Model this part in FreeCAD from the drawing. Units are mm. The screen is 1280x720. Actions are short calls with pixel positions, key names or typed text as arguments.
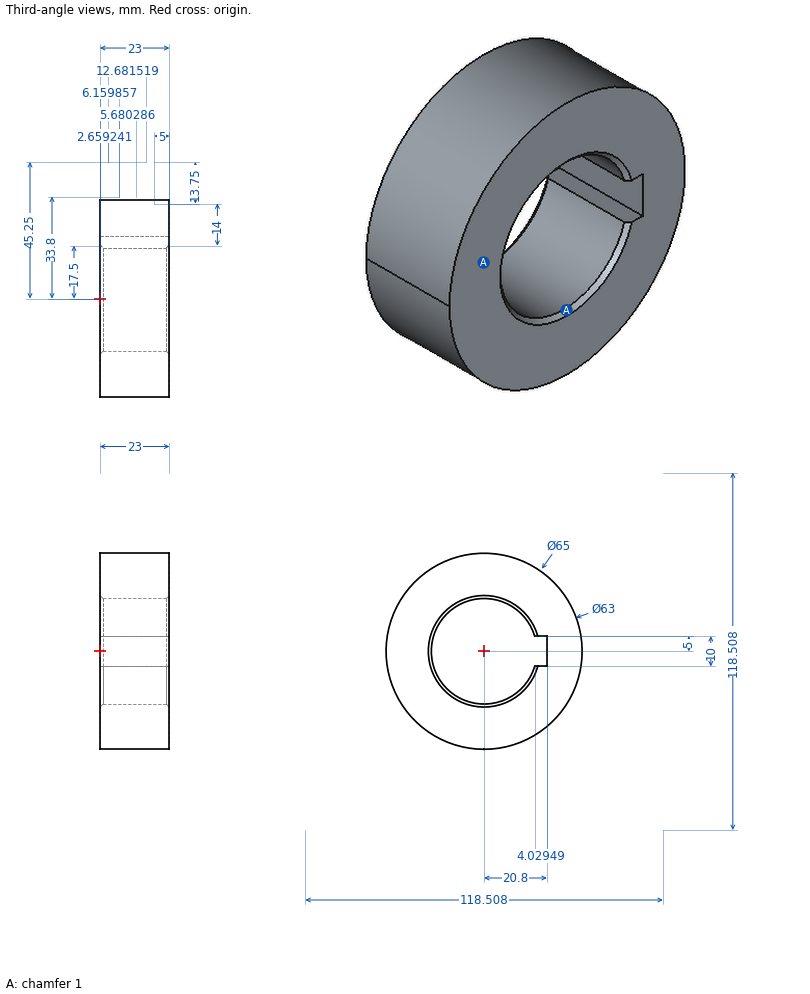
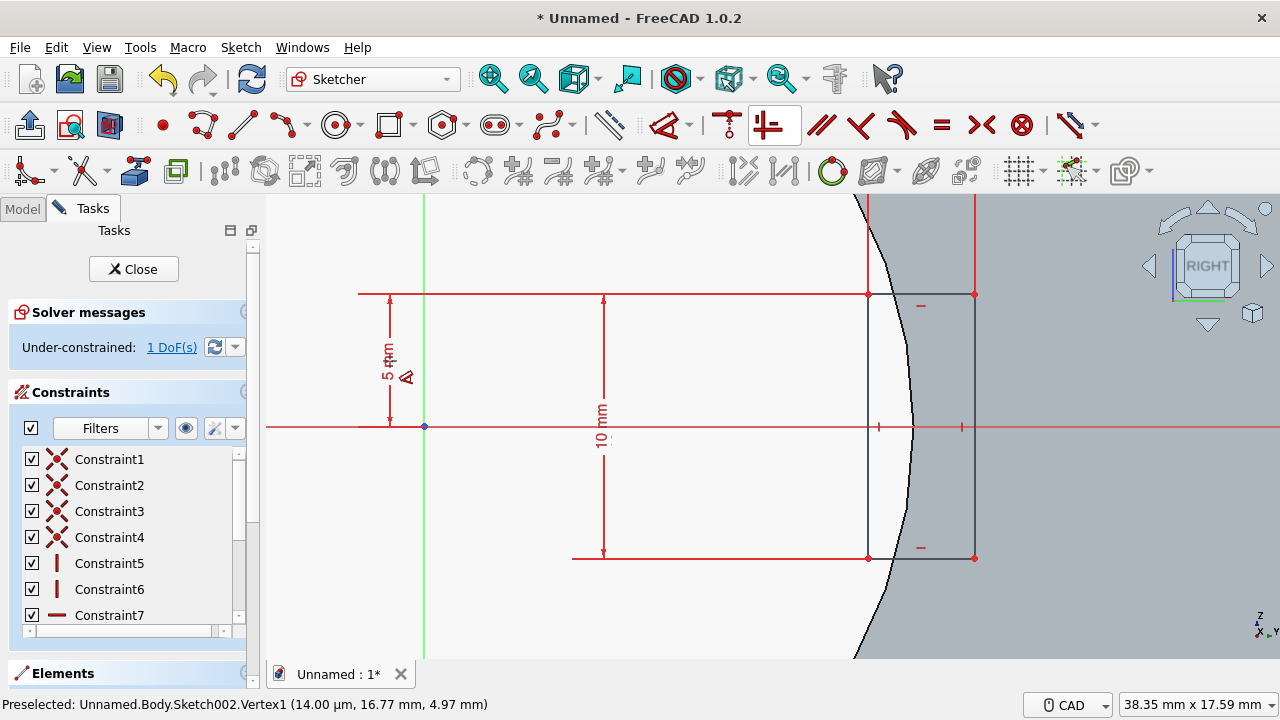
click(975, 559)
click(699, 593)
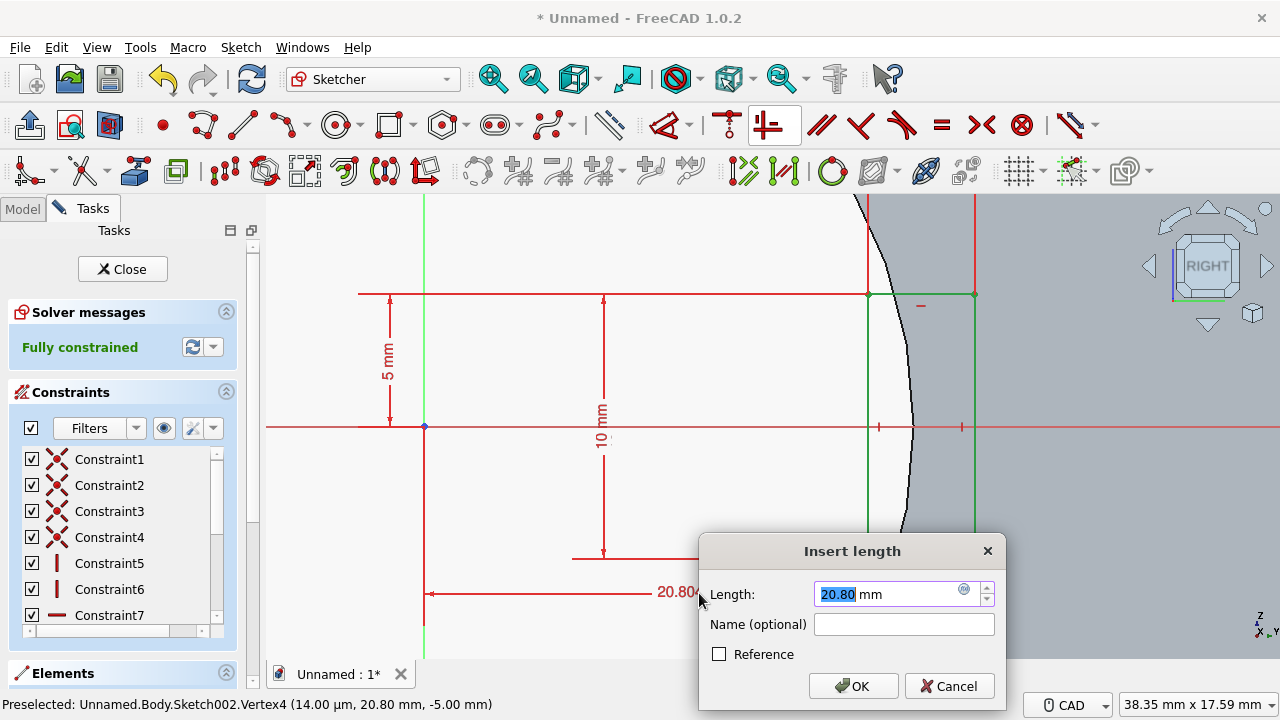
text(20.8)
key(Return)
key(Escape)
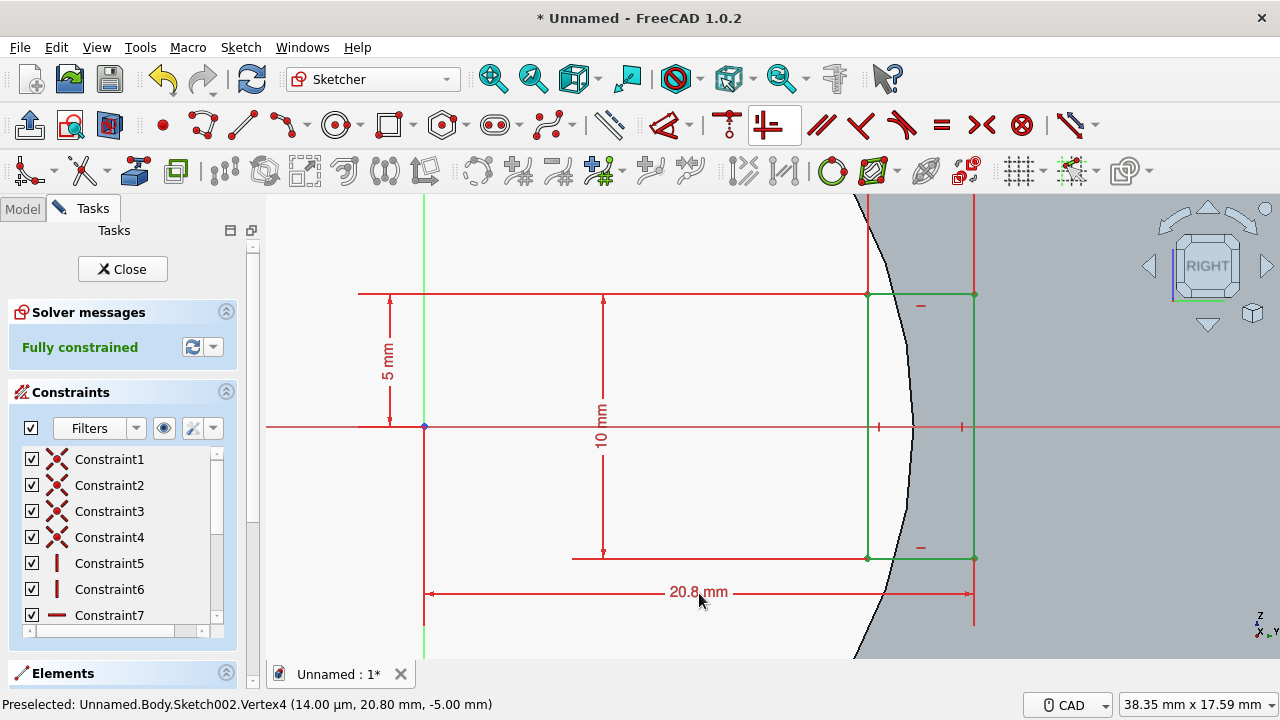
click(123, 269)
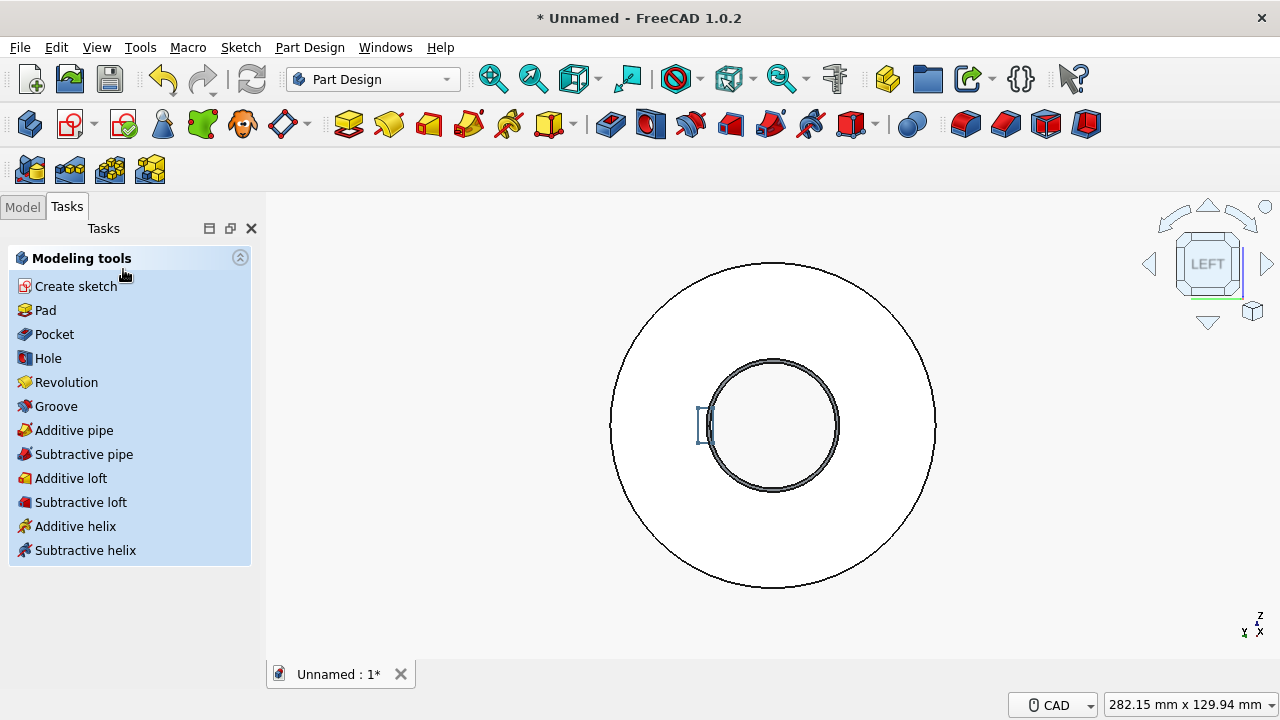
click(612, 124)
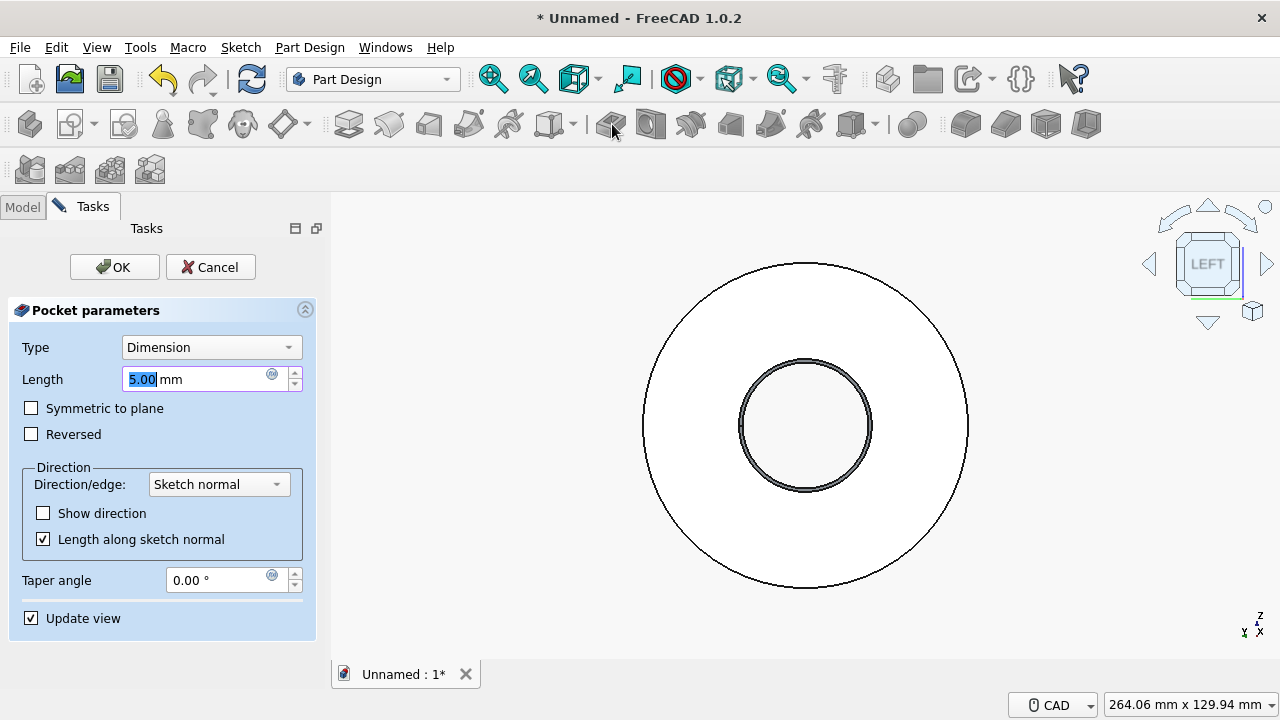
click(212, 348)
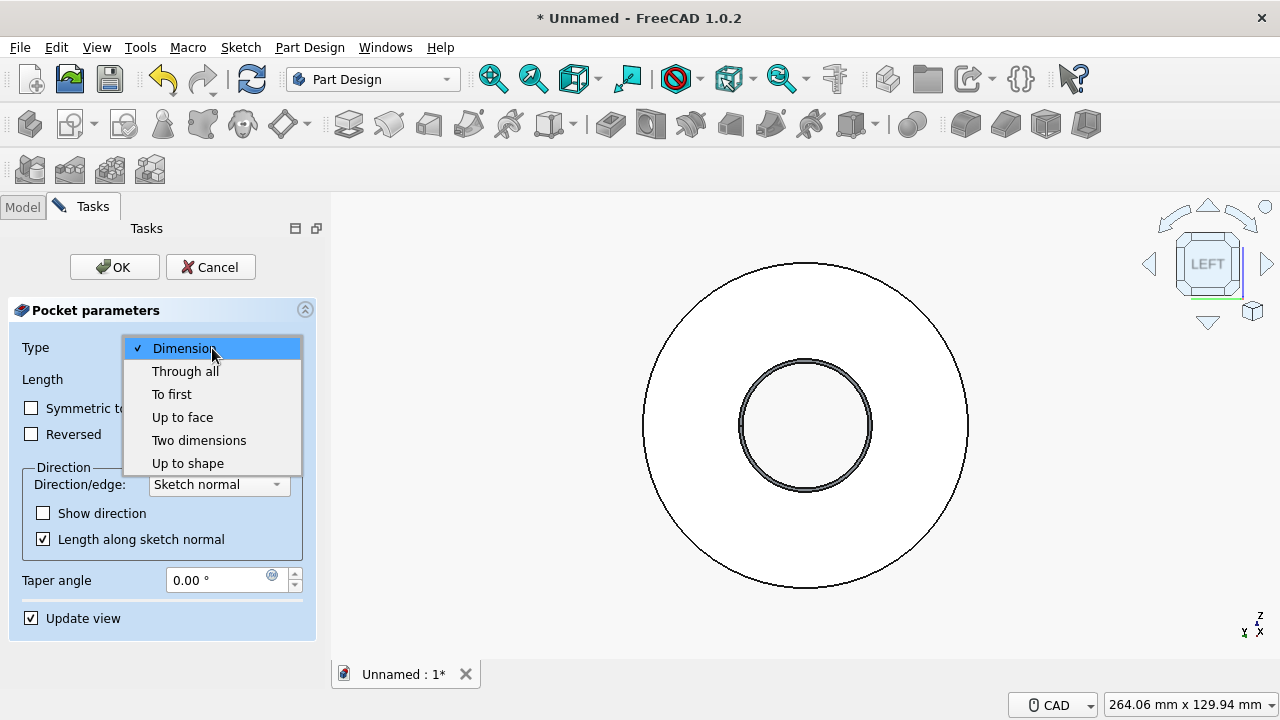
click(212, 372)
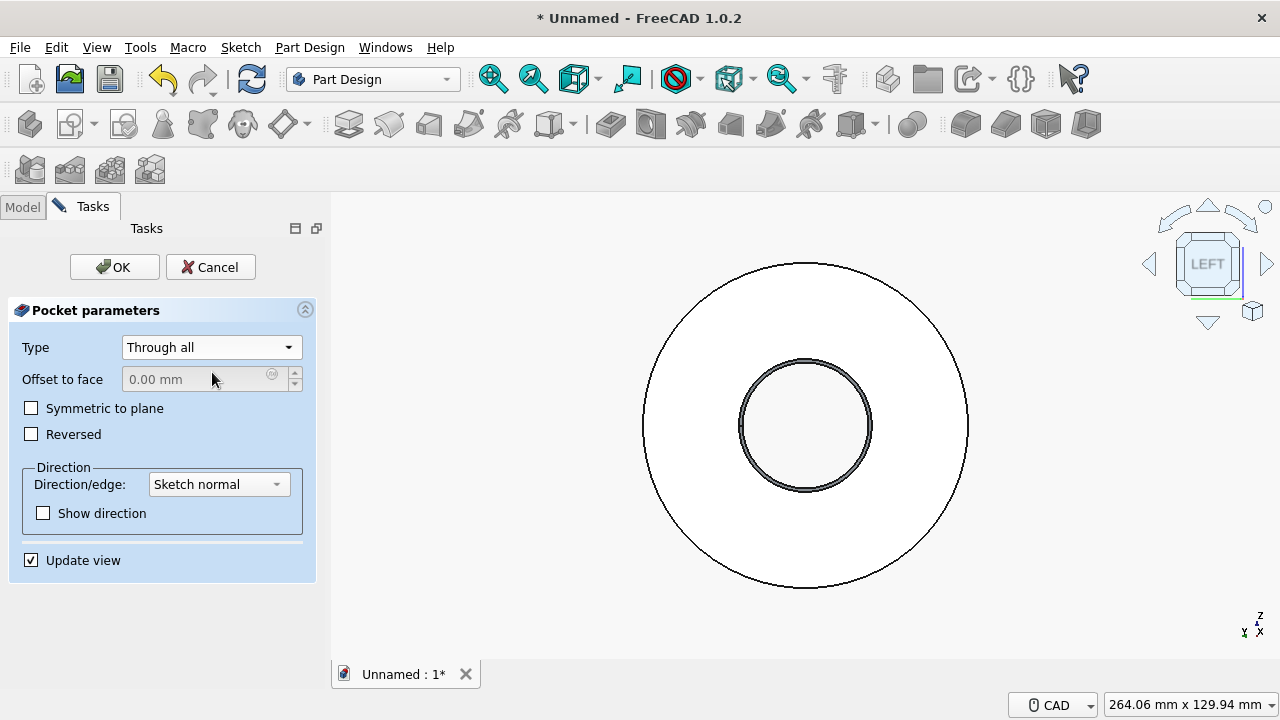
click(30, 434)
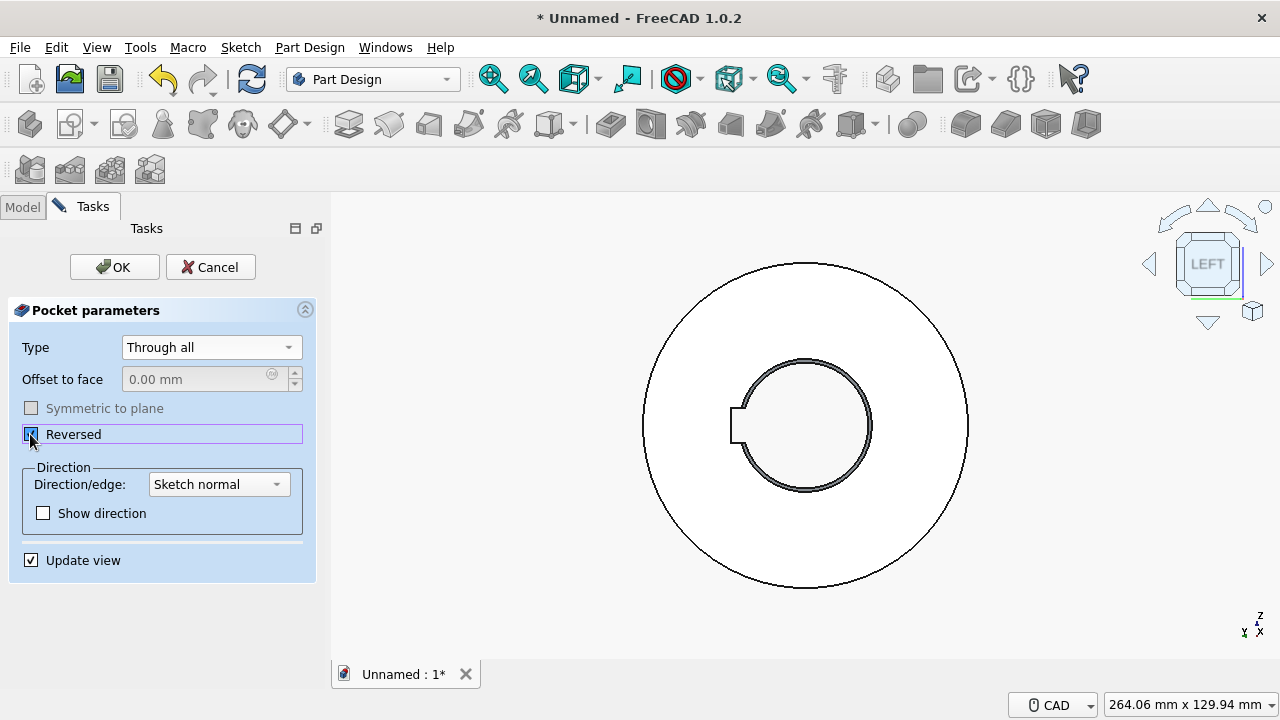
click(115, 267)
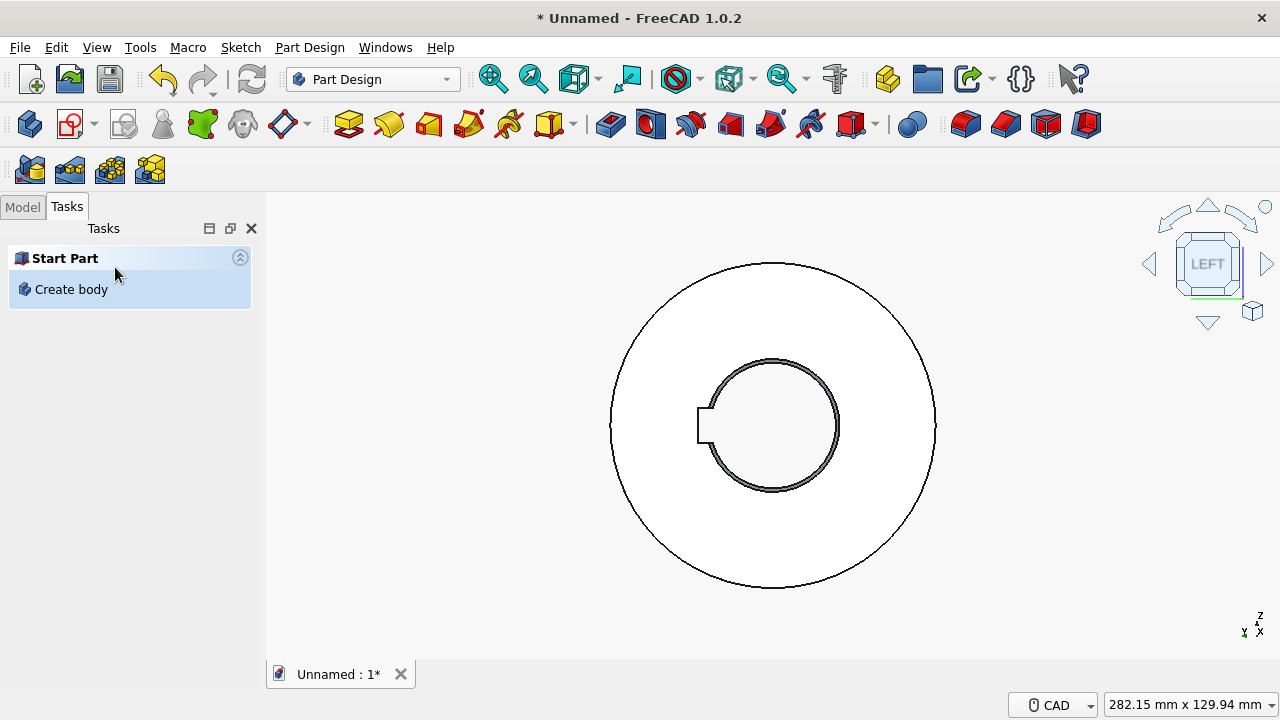
click(70, 124)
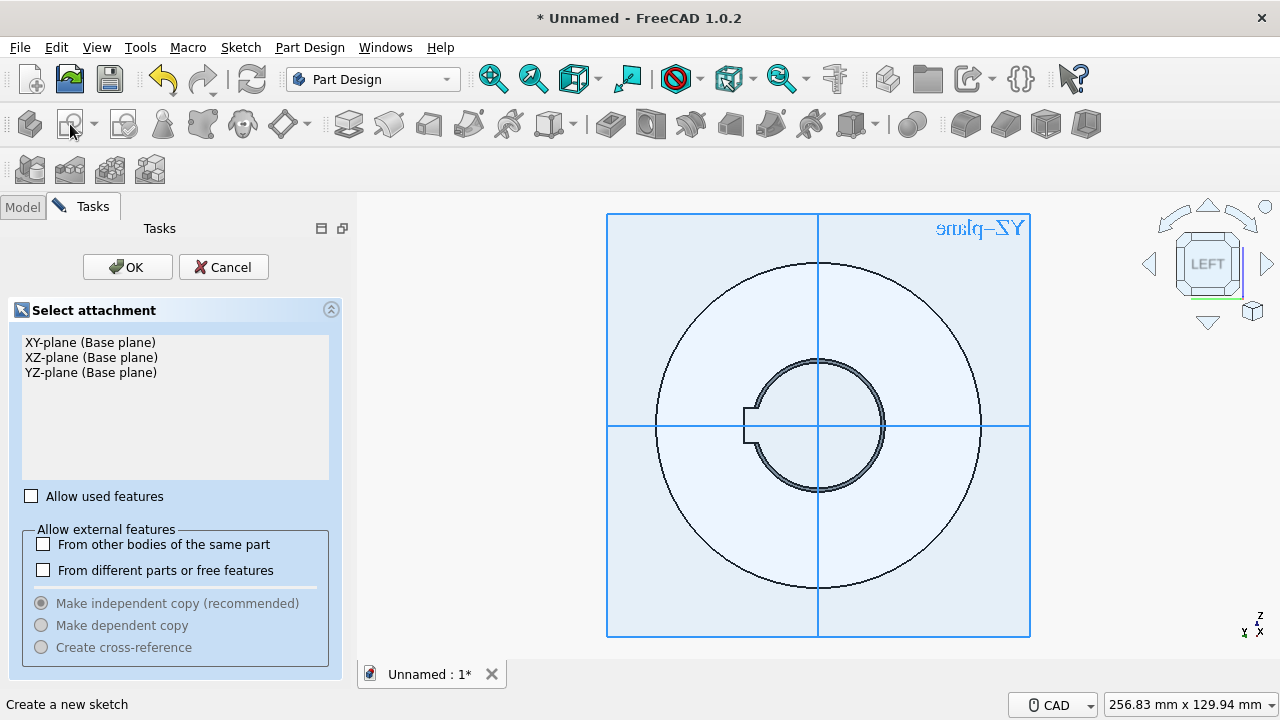
click(82, 372)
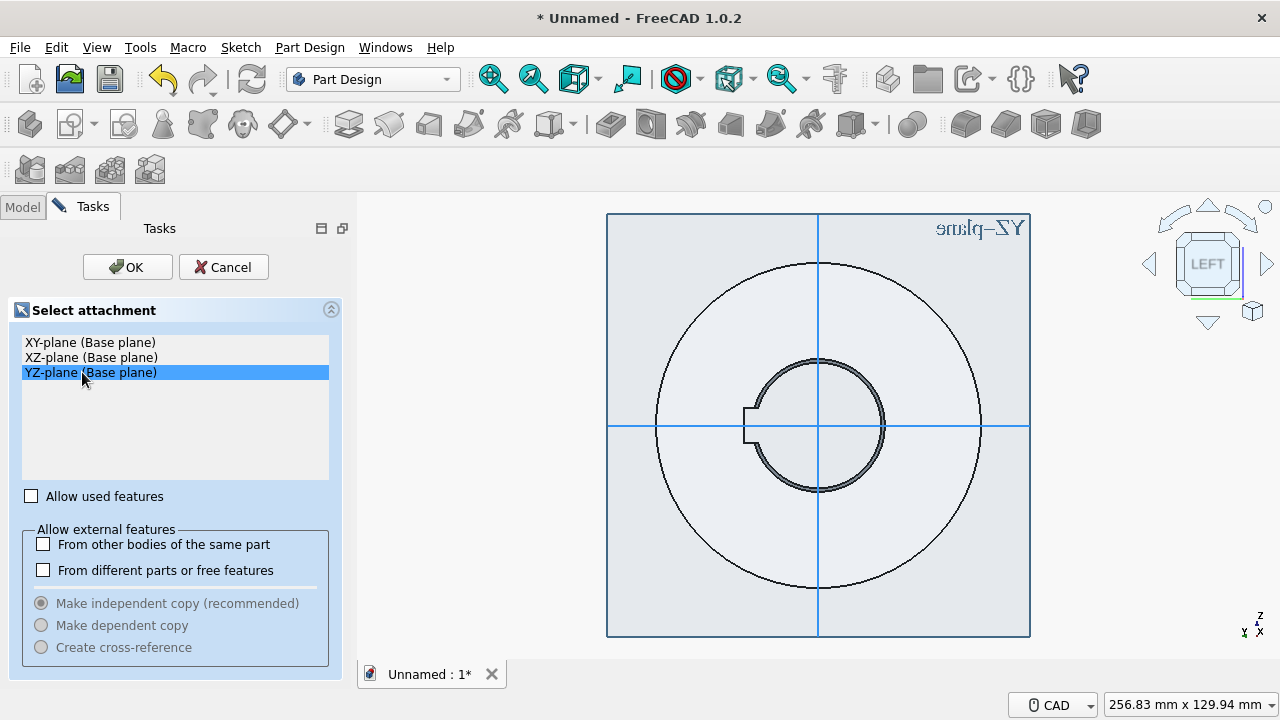
click(128, 267)